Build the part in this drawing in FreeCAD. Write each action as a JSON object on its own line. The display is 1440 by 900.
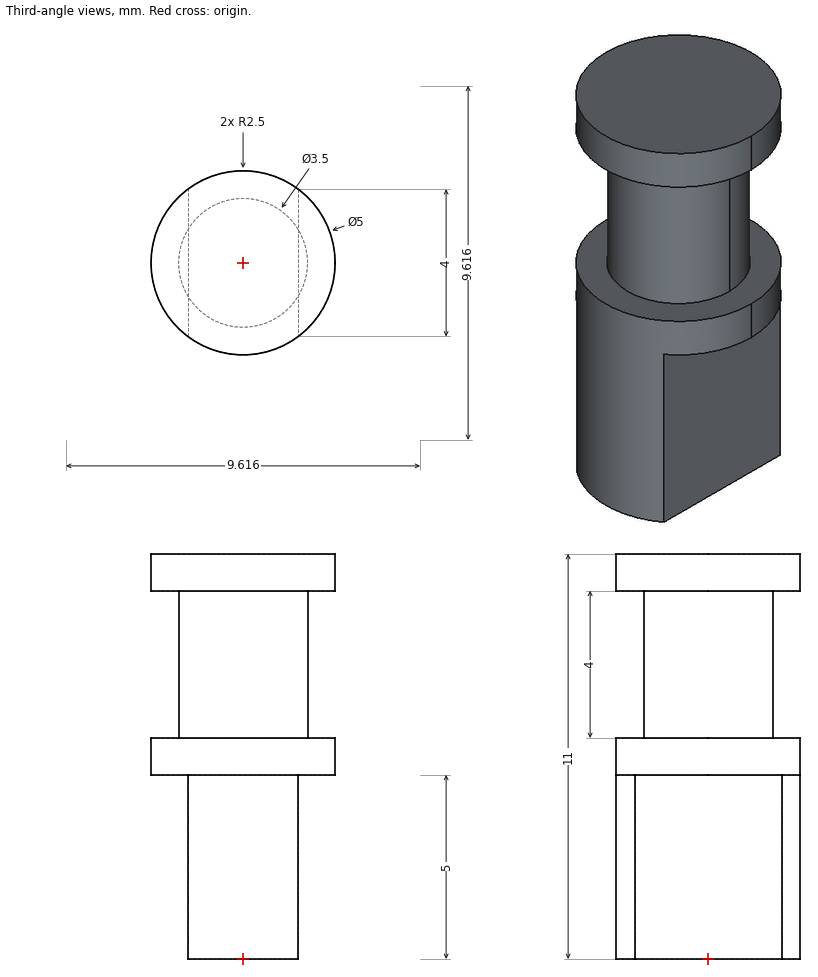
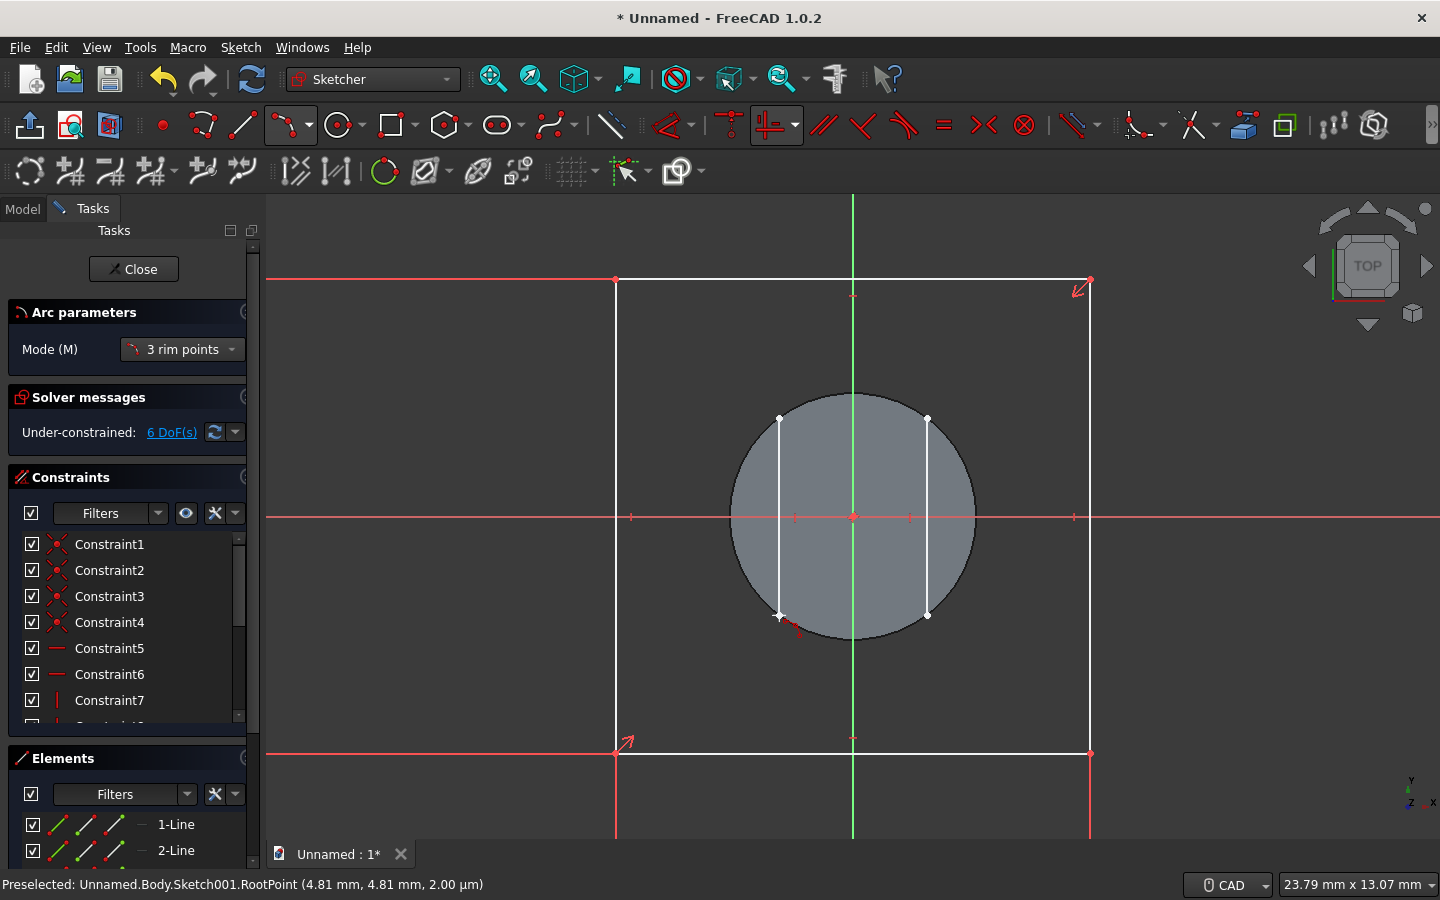
{"action": "left_click", "coordinate": [927, 419]}
{"action": "left_click", "coordinate": [779, 419]}
{"action": "left_click", "coordinate": [869, 394]}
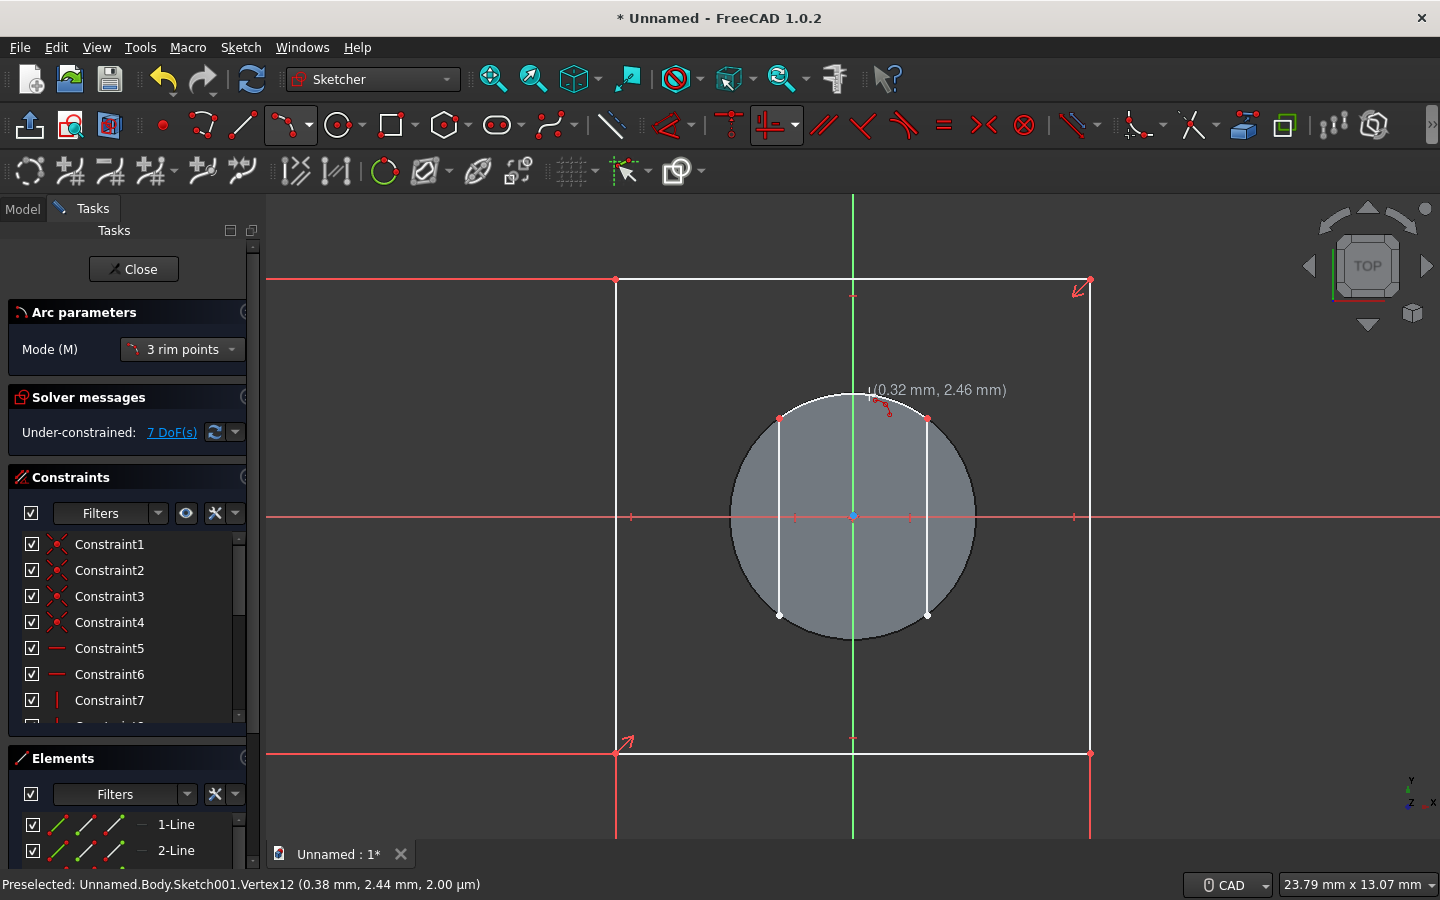
{"action": "left_click", "coordinate": [779, 616]}
{"action": "left_click", "coordinate": [927, 616]}
{"action": "left_click", "coordinate": [837, 639]}
{"action": "key", "text": "Escape"}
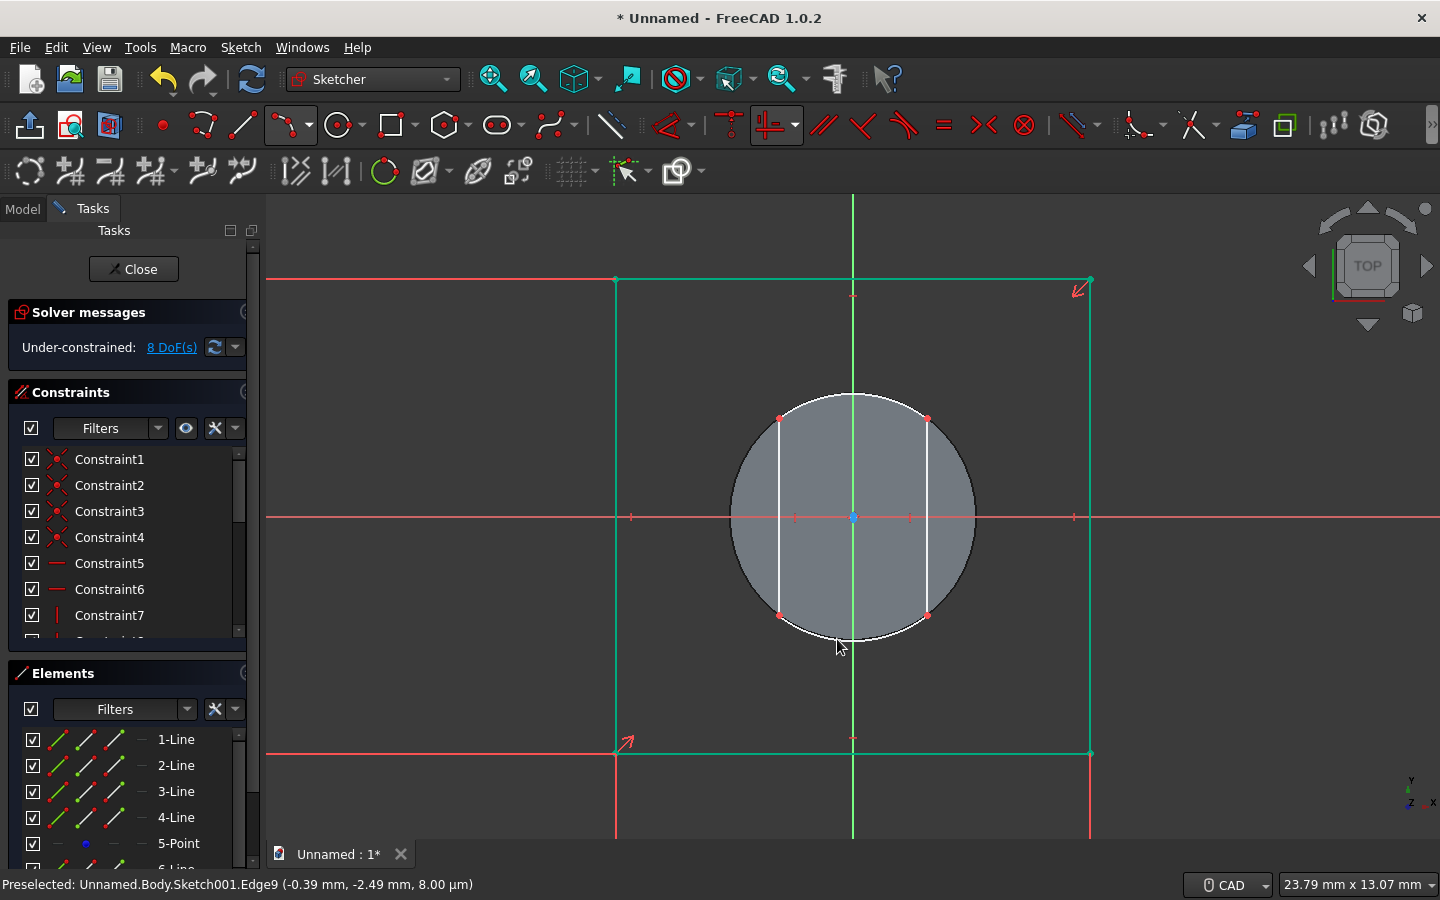
{"action": "left_click", "coordinate": [884, 398]}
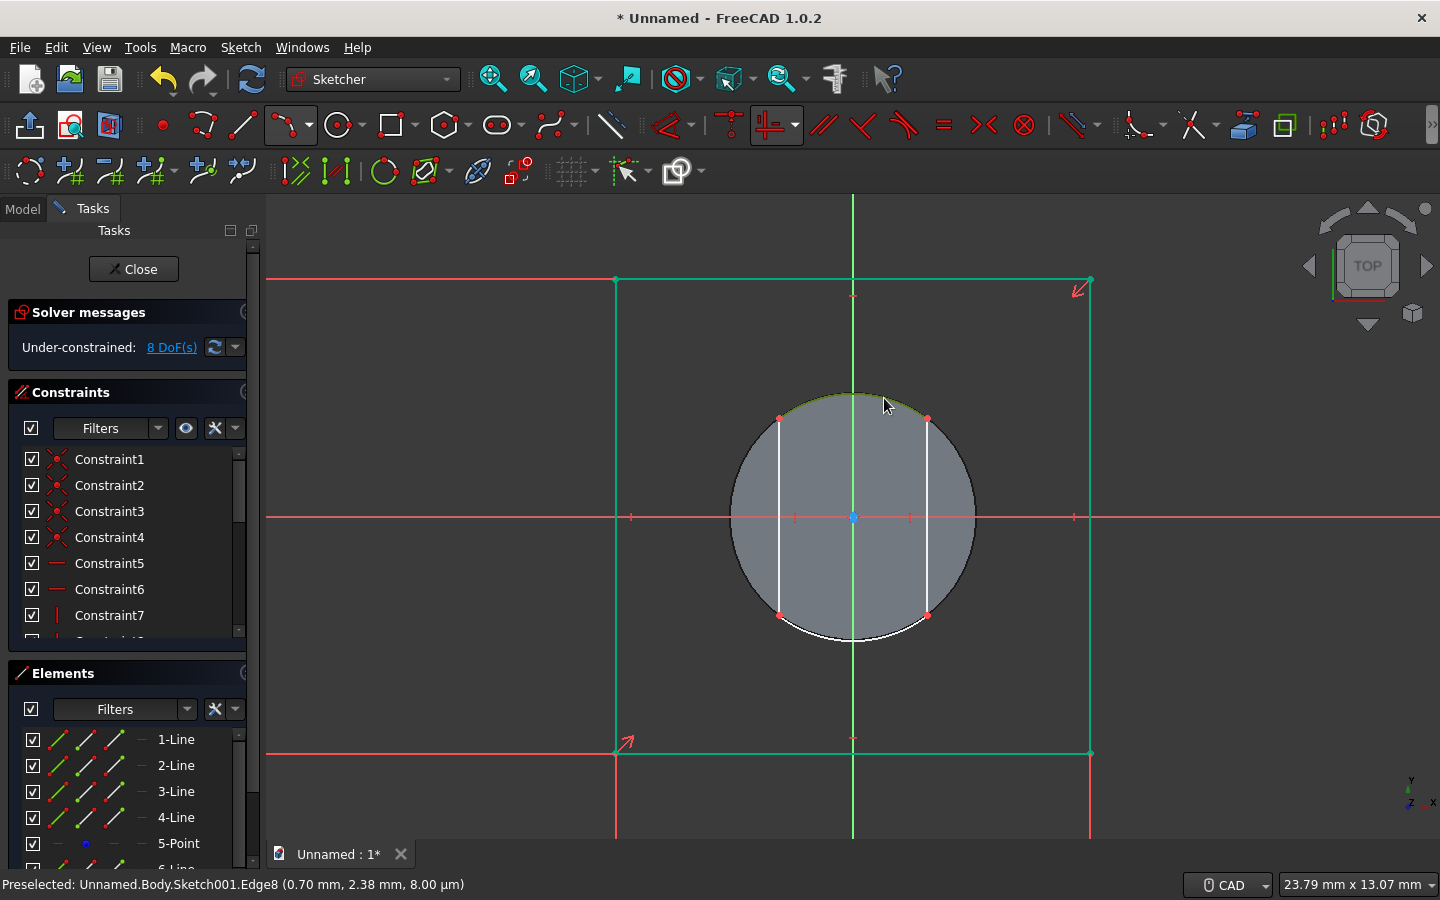
{"action": "left_click", "coordinate": [822, 637]}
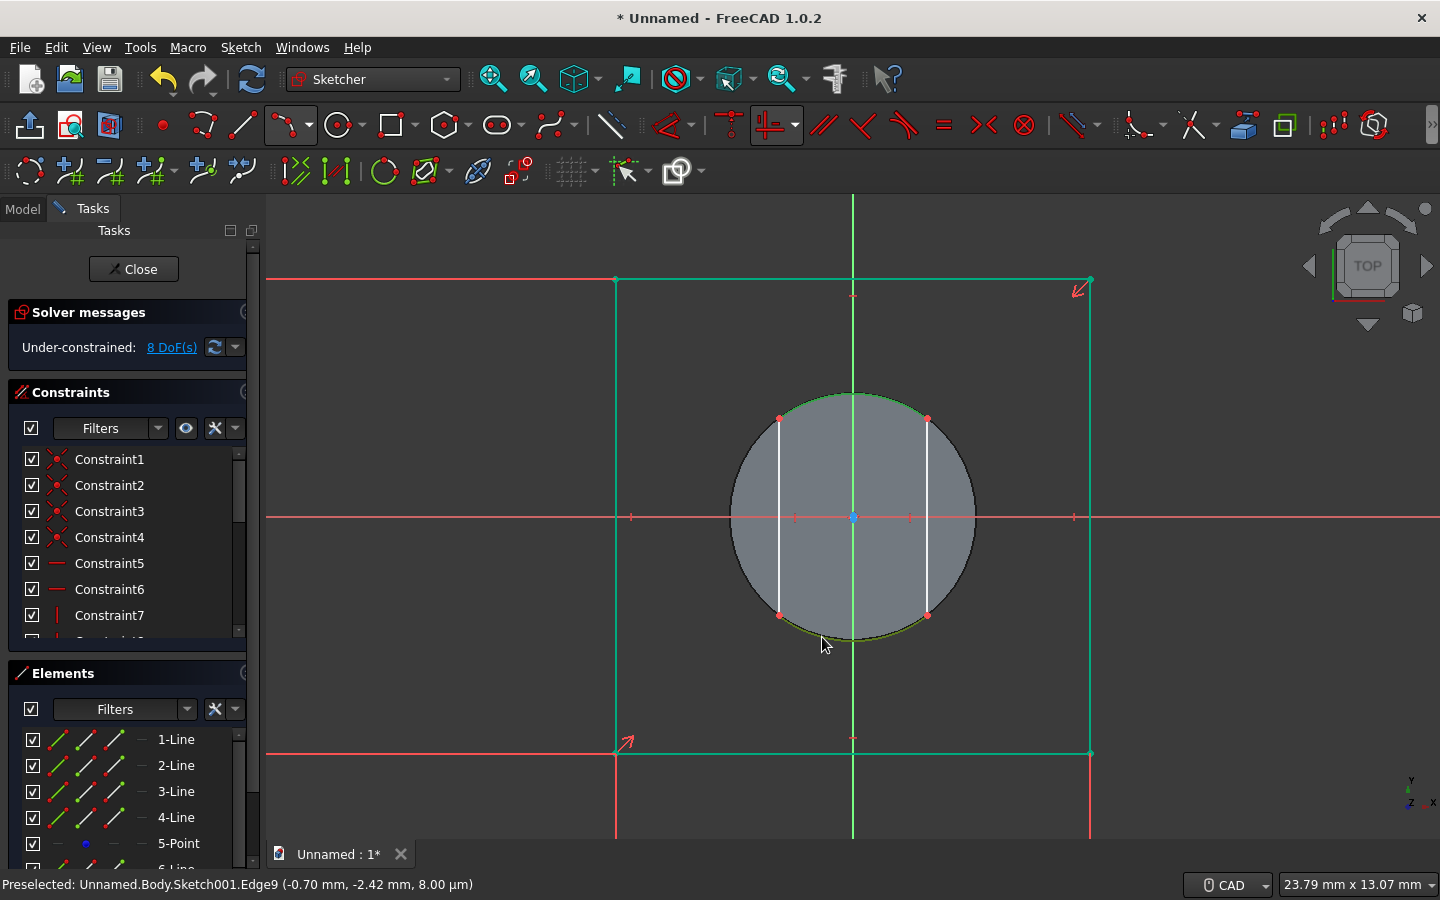
{"action": "key", "text": "c"}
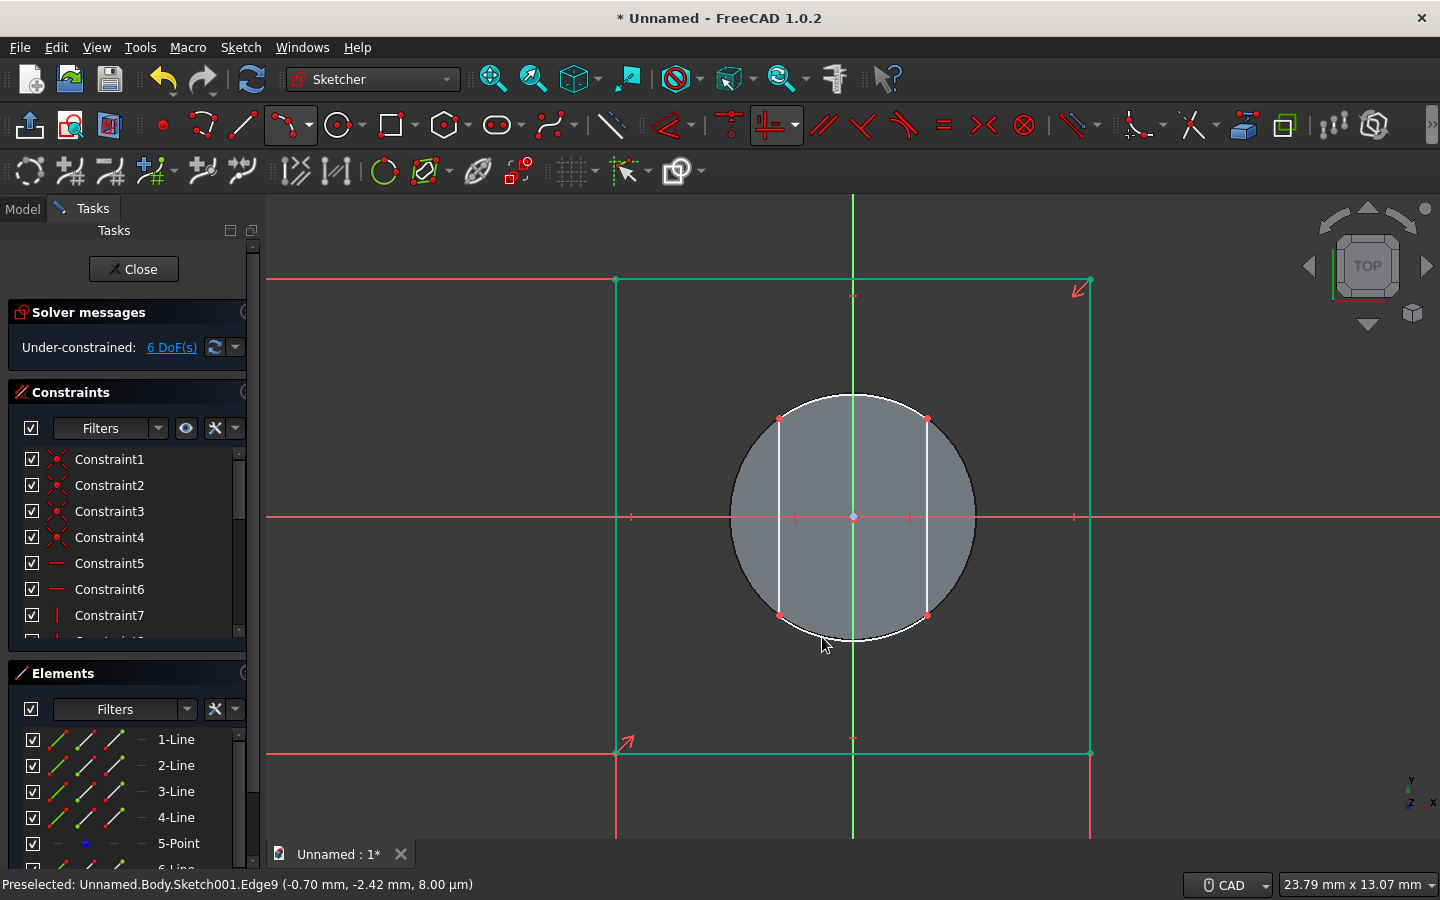
{"action": "left_click_drag", "start_coordinate": [843, 506], "coordinate": [863, 529]}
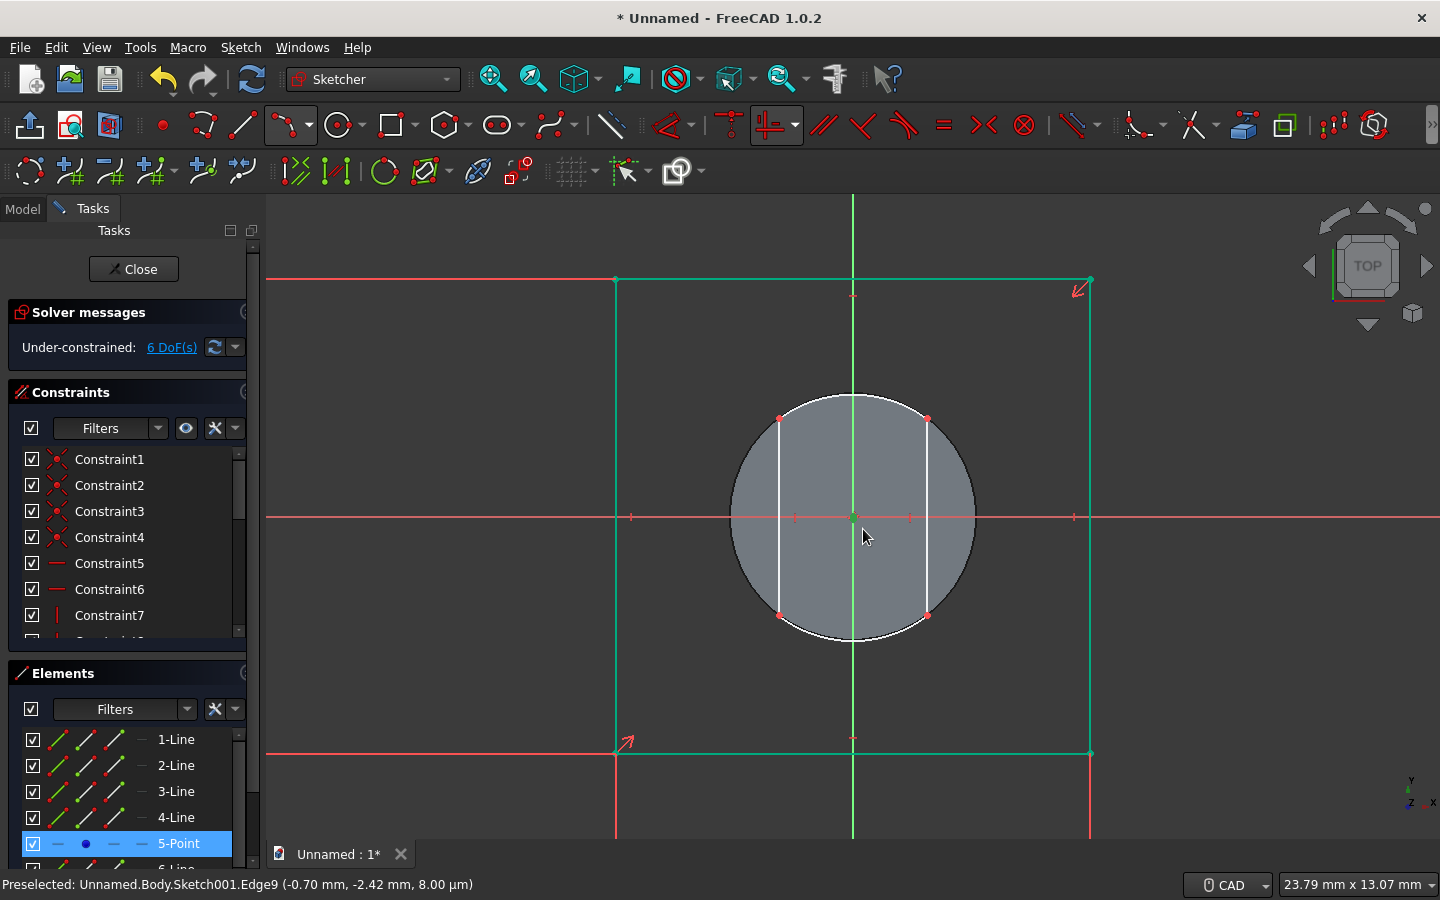
{"action": "left_click", "coordinate": [730, 126]}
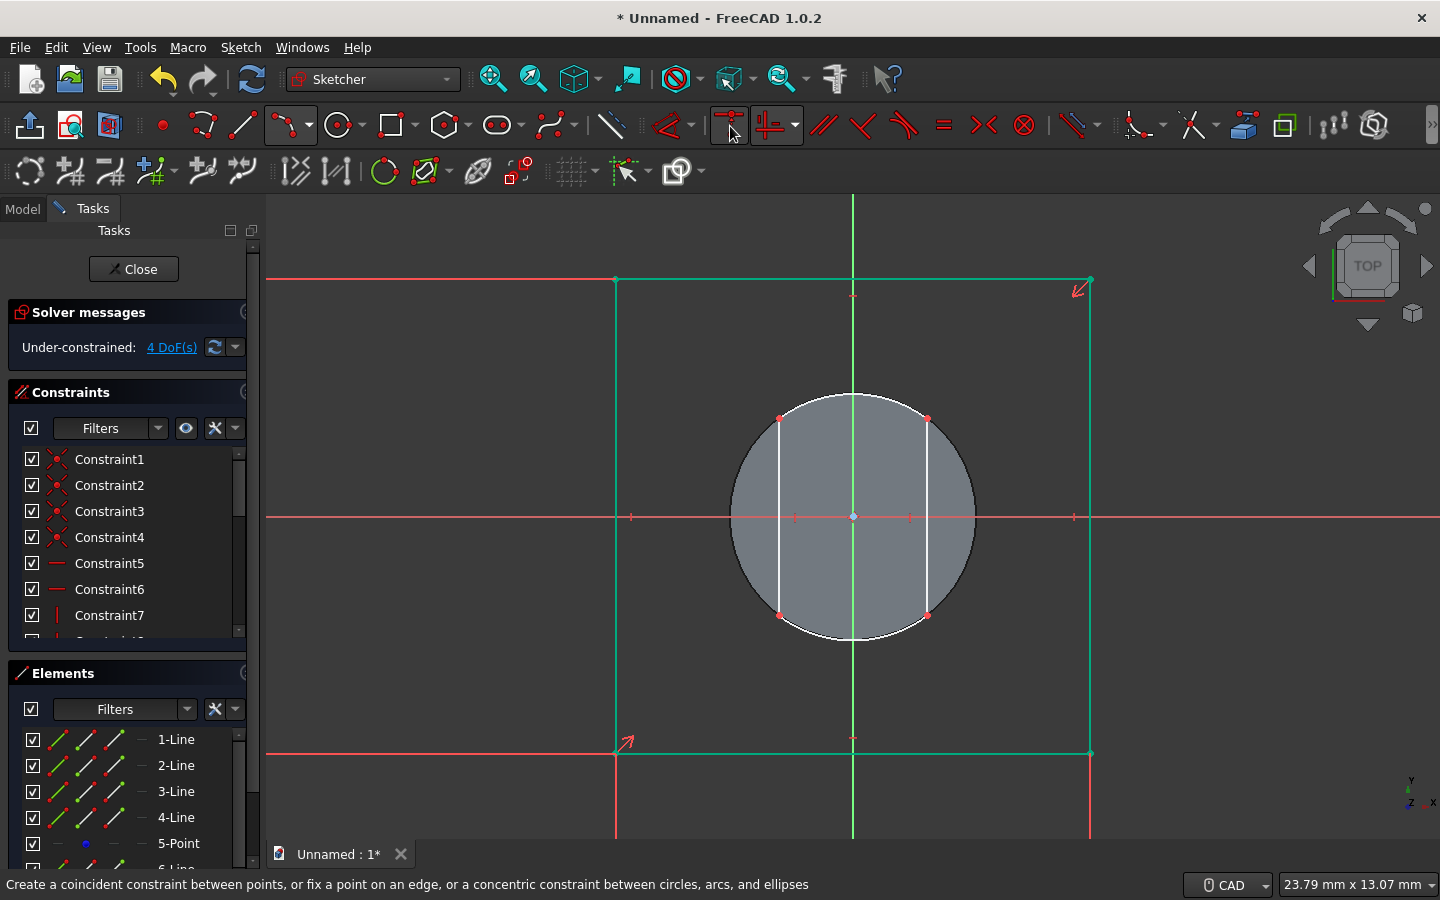
{"action": "left_click", "coordinate": [884, 398]}